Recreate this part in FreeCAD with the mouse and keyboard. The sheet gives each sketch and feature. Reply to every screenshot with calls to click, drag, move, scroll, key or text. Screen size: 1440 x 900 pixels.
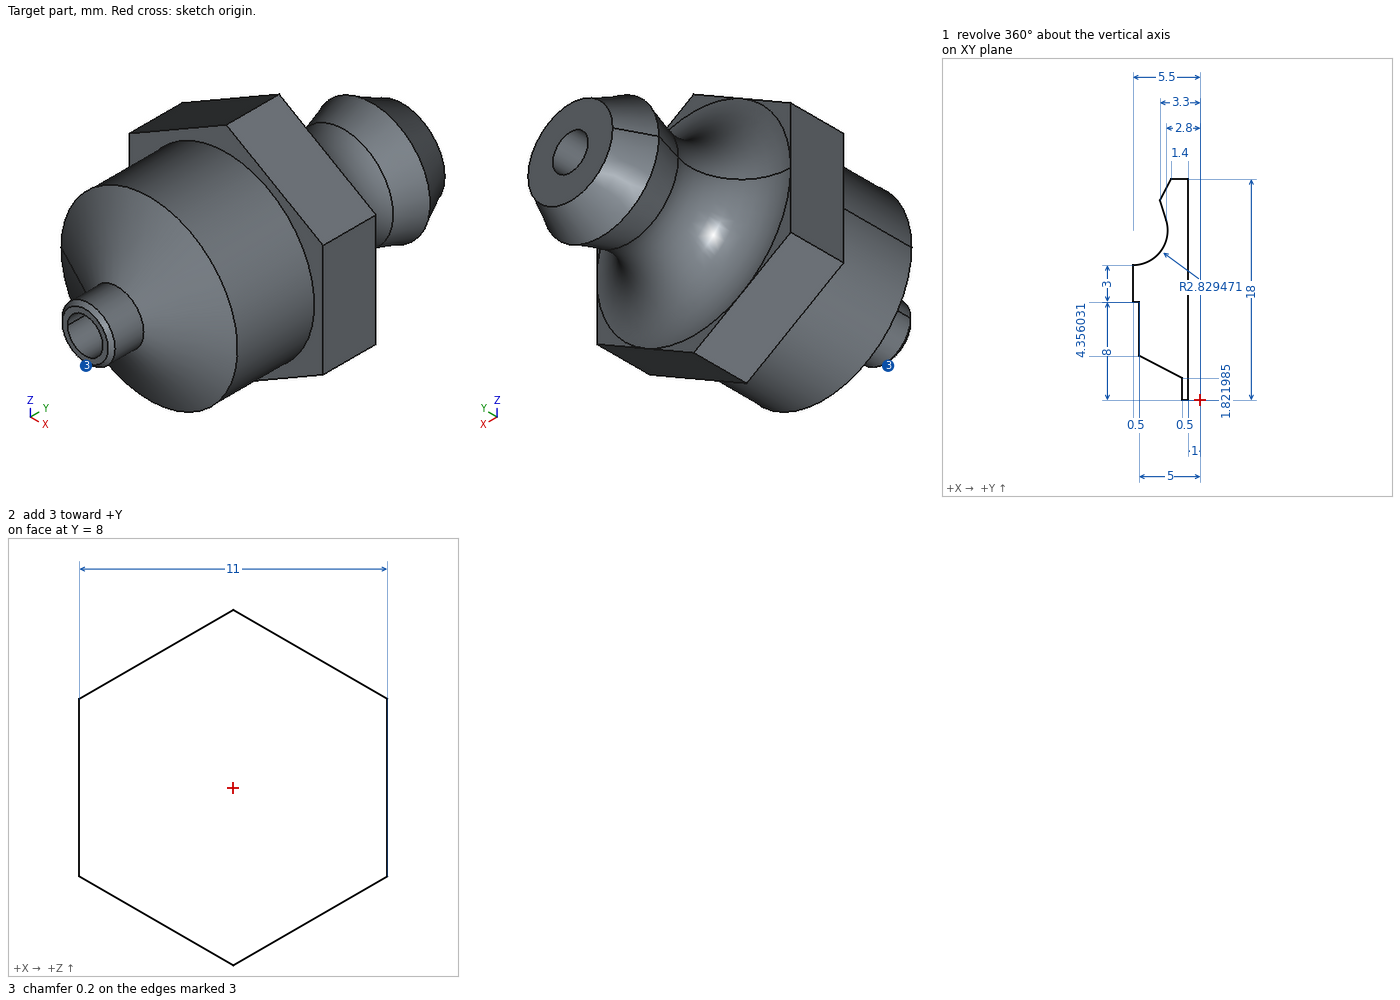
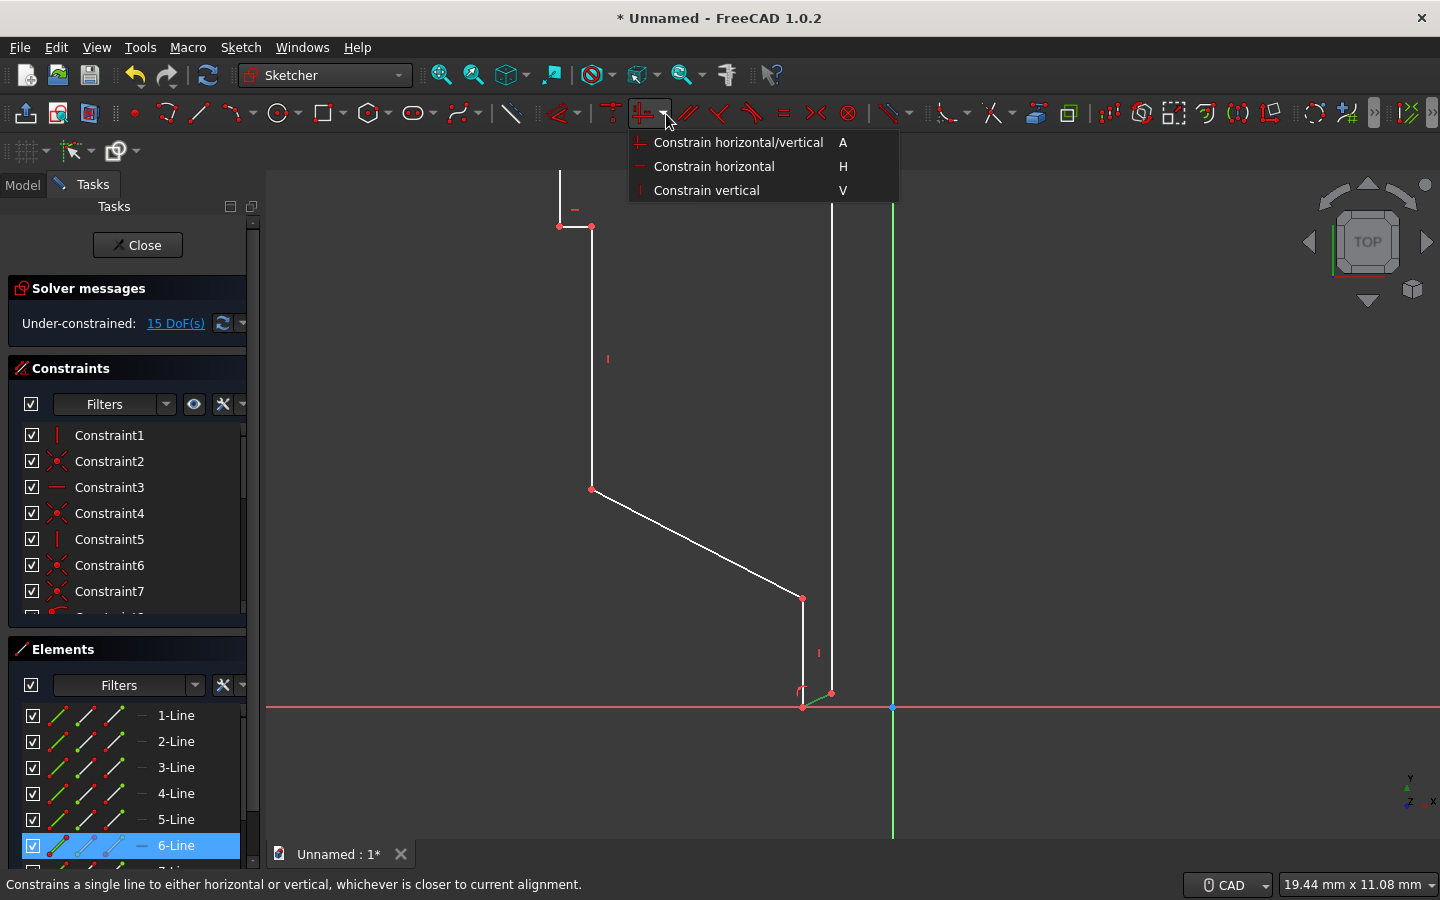
click(764, 166)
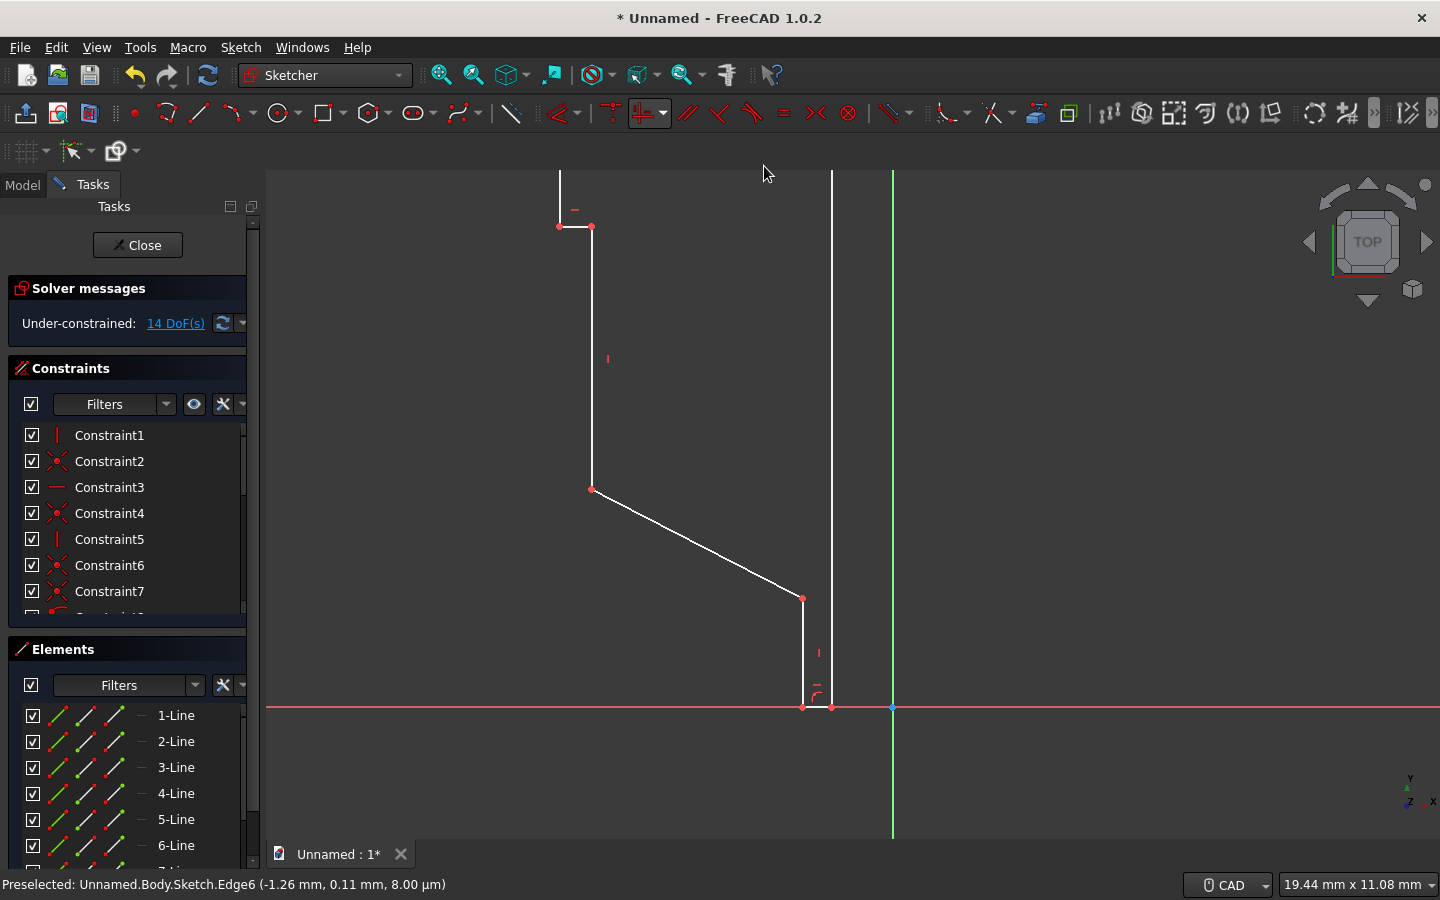
scroll(818, 703, down, 5)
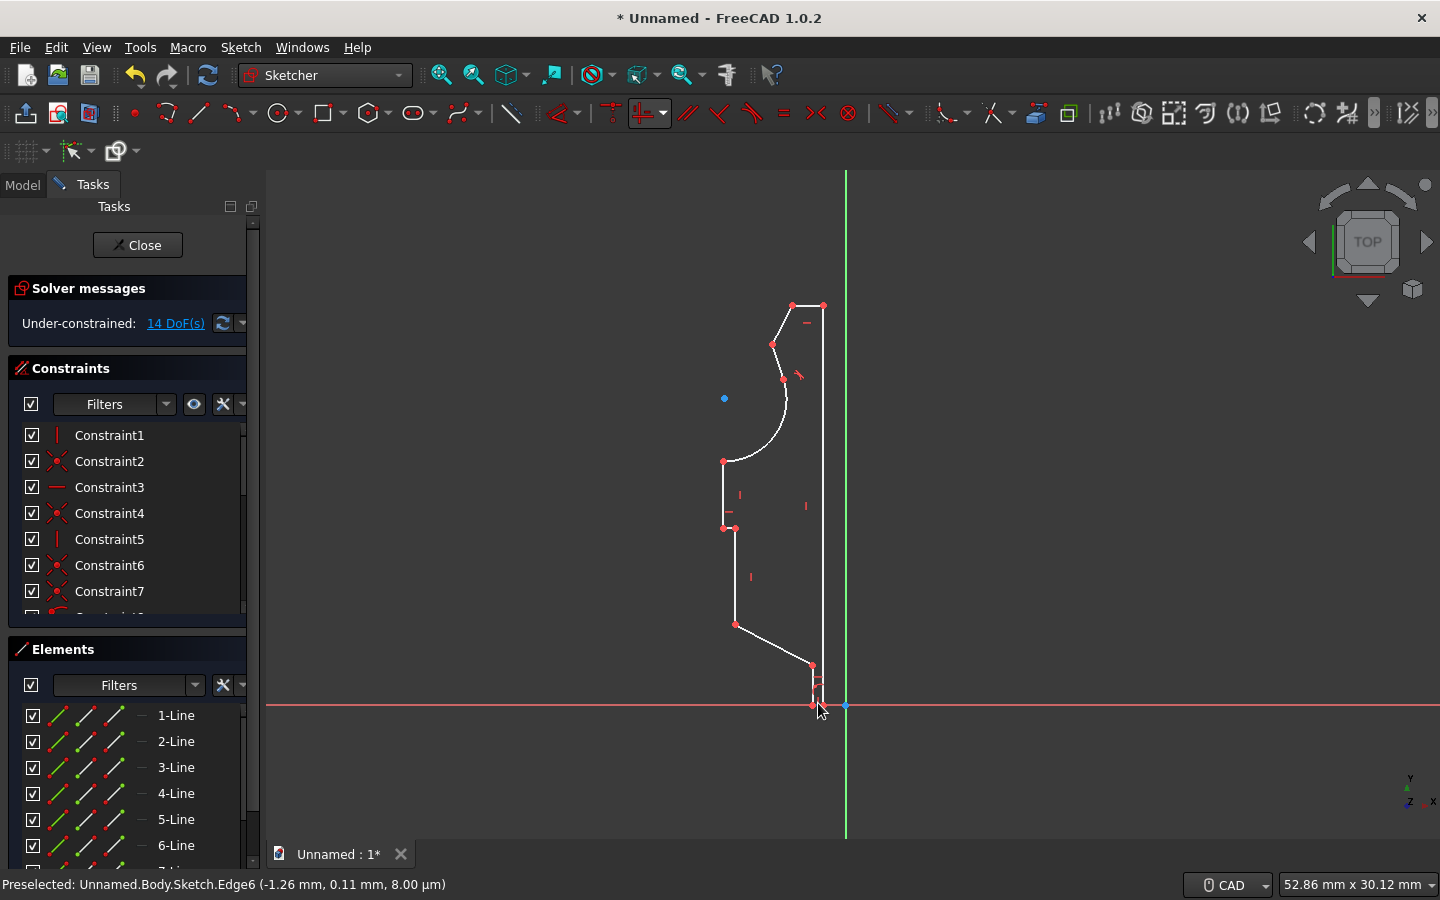
click(757, 452)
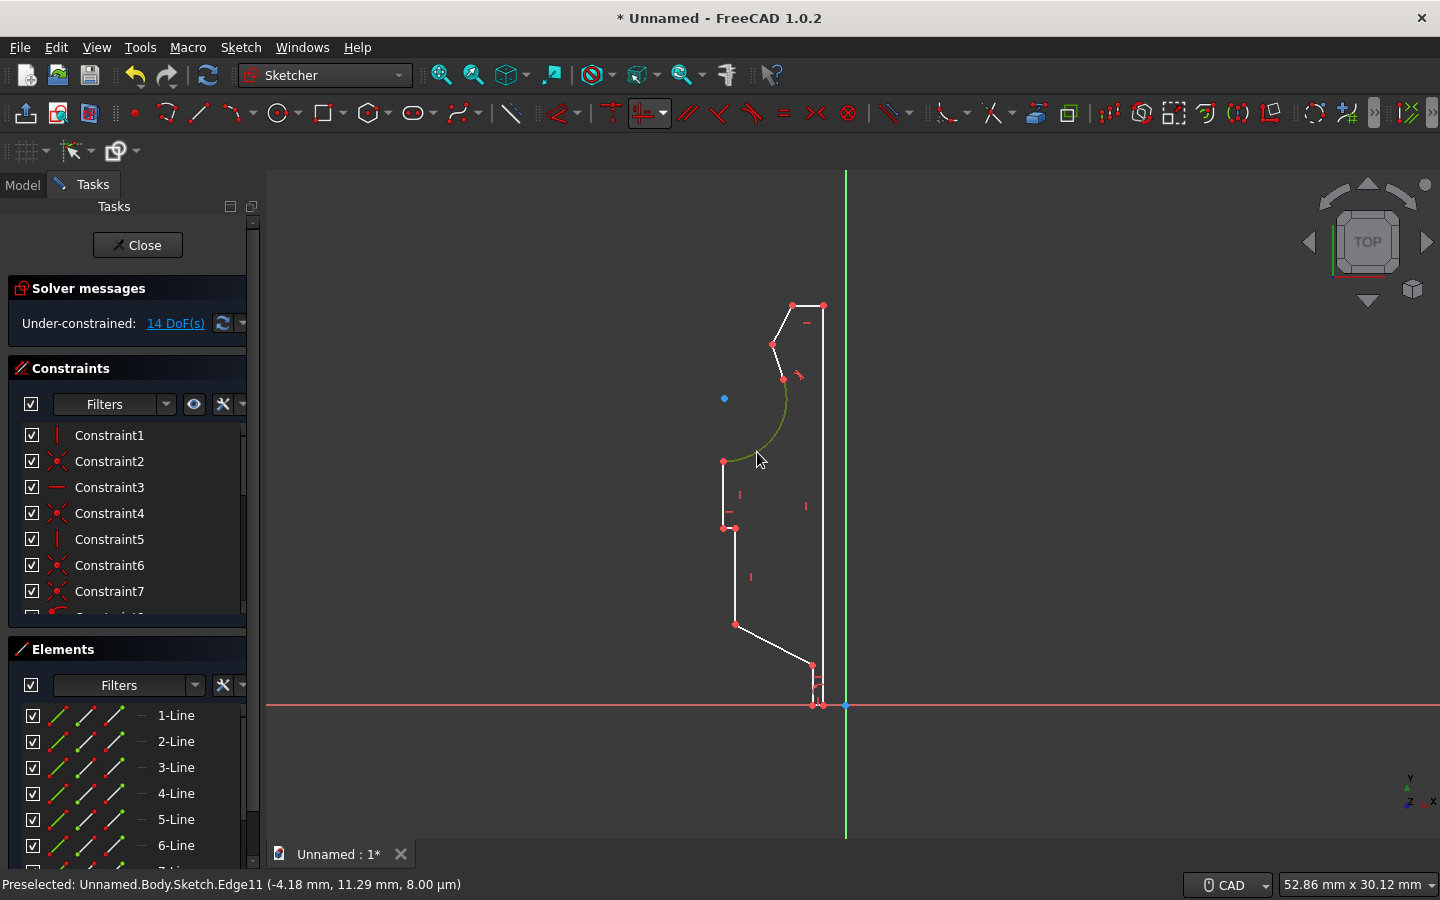
click(580, 114)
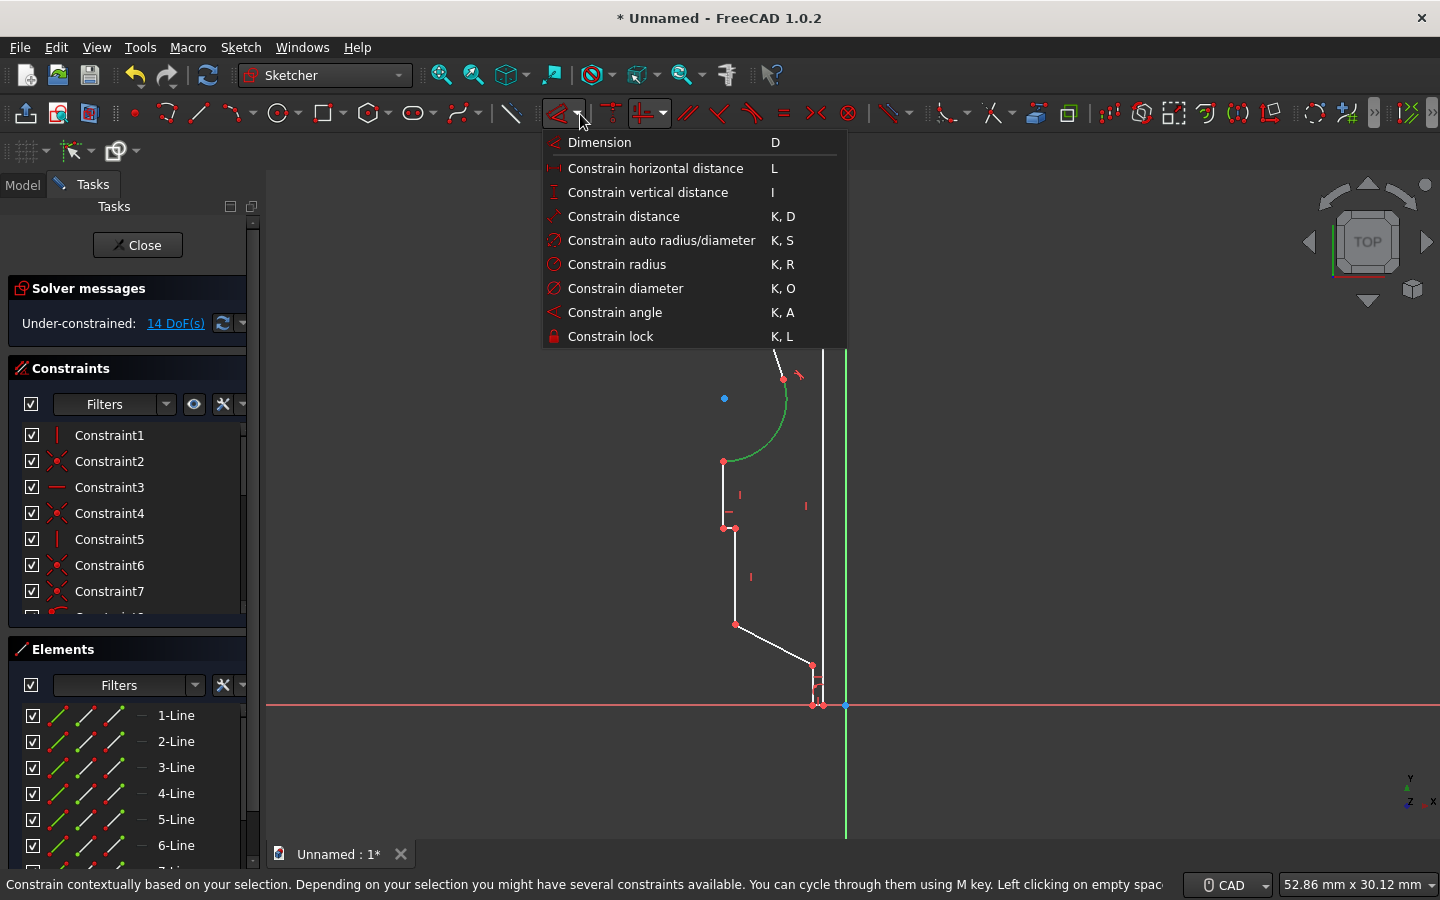
click(695, 264)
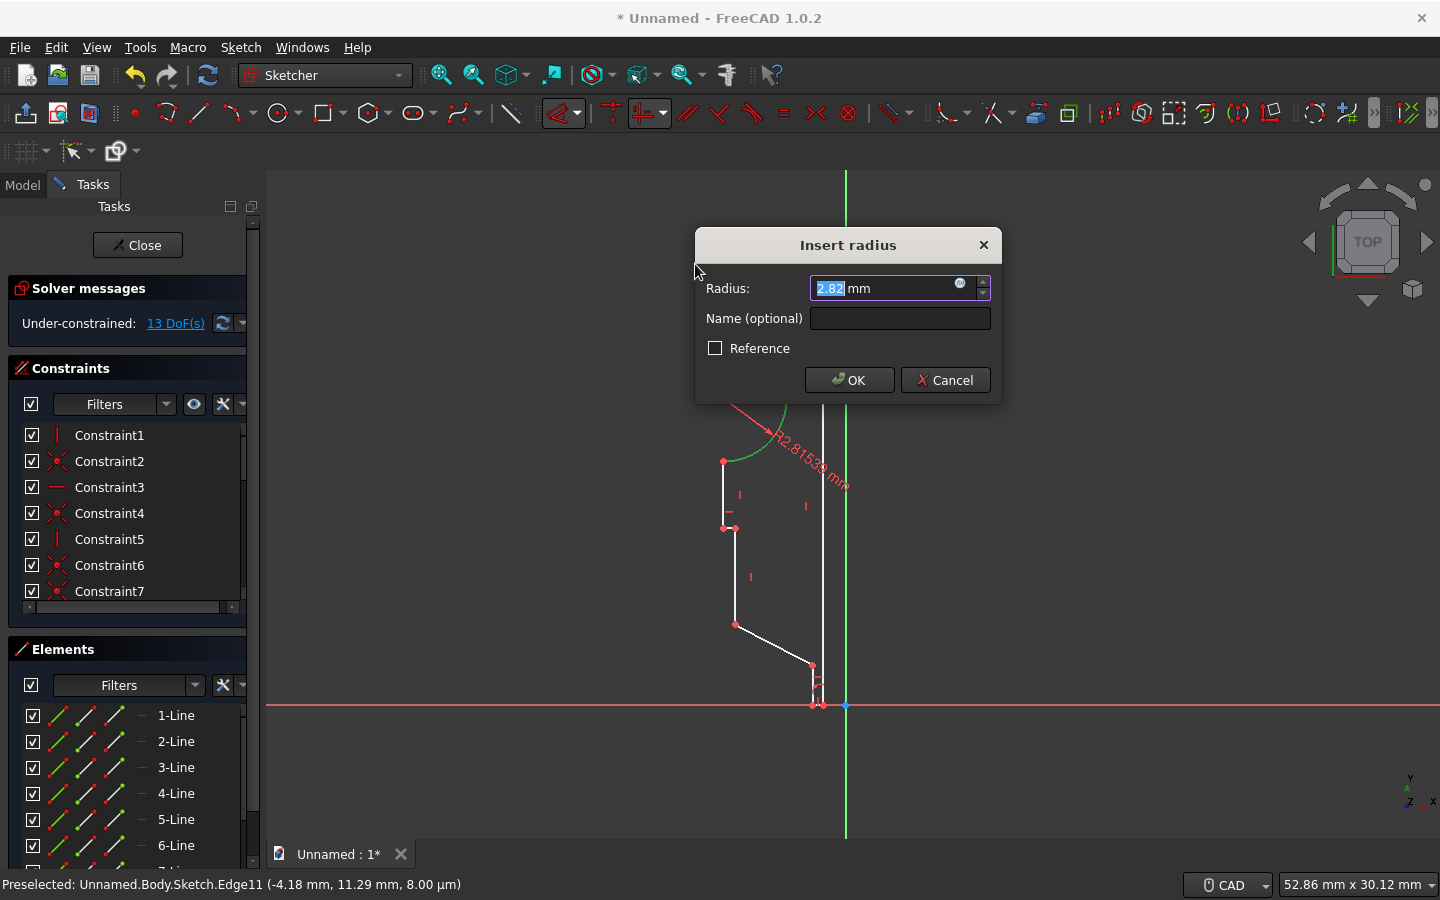
text(2.829471)
key(Return)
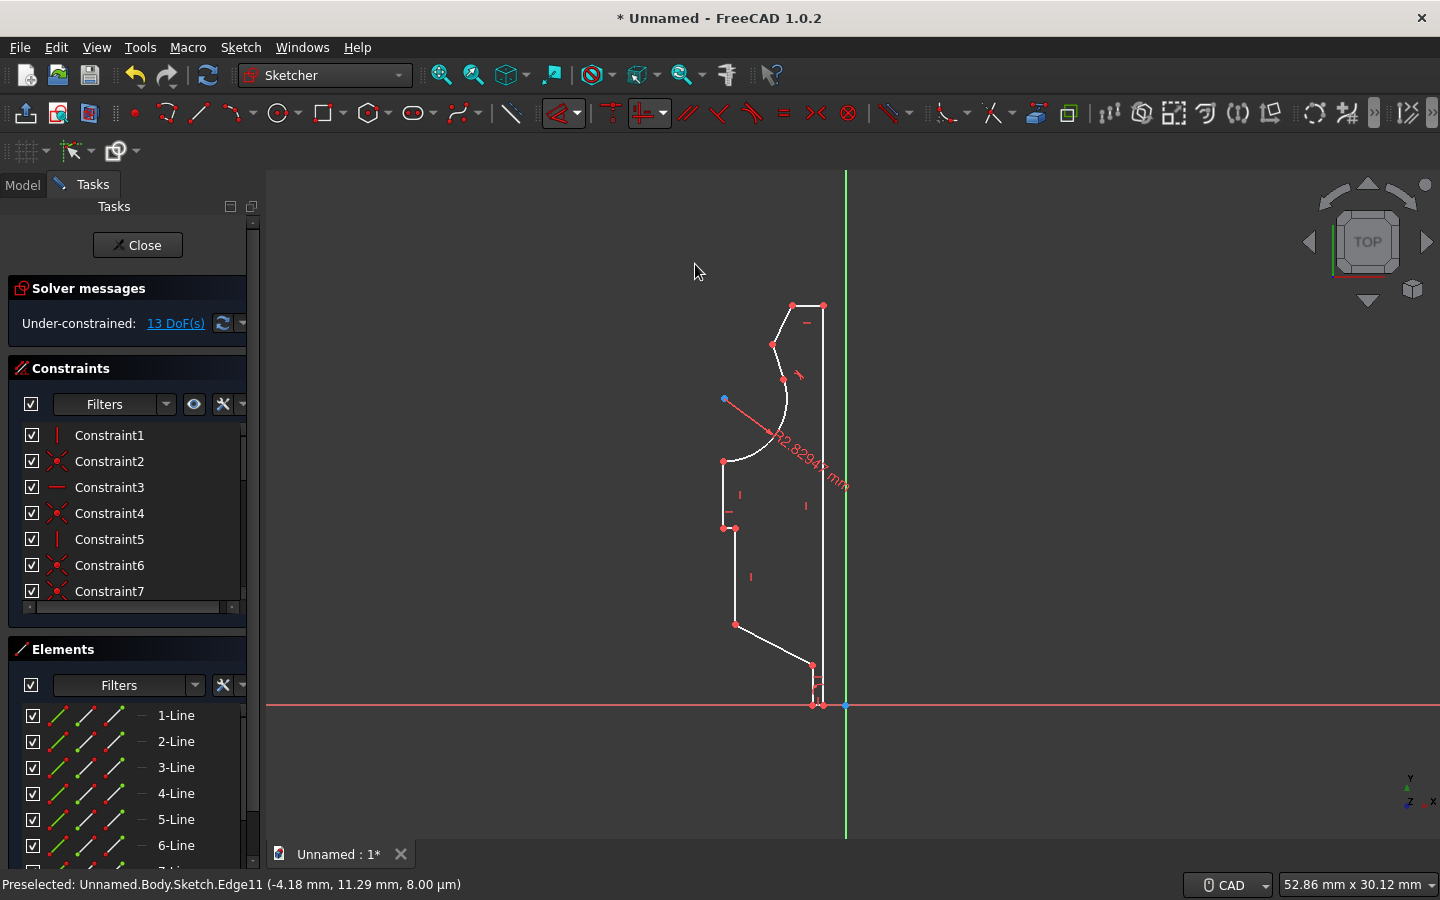
click(723, 481)